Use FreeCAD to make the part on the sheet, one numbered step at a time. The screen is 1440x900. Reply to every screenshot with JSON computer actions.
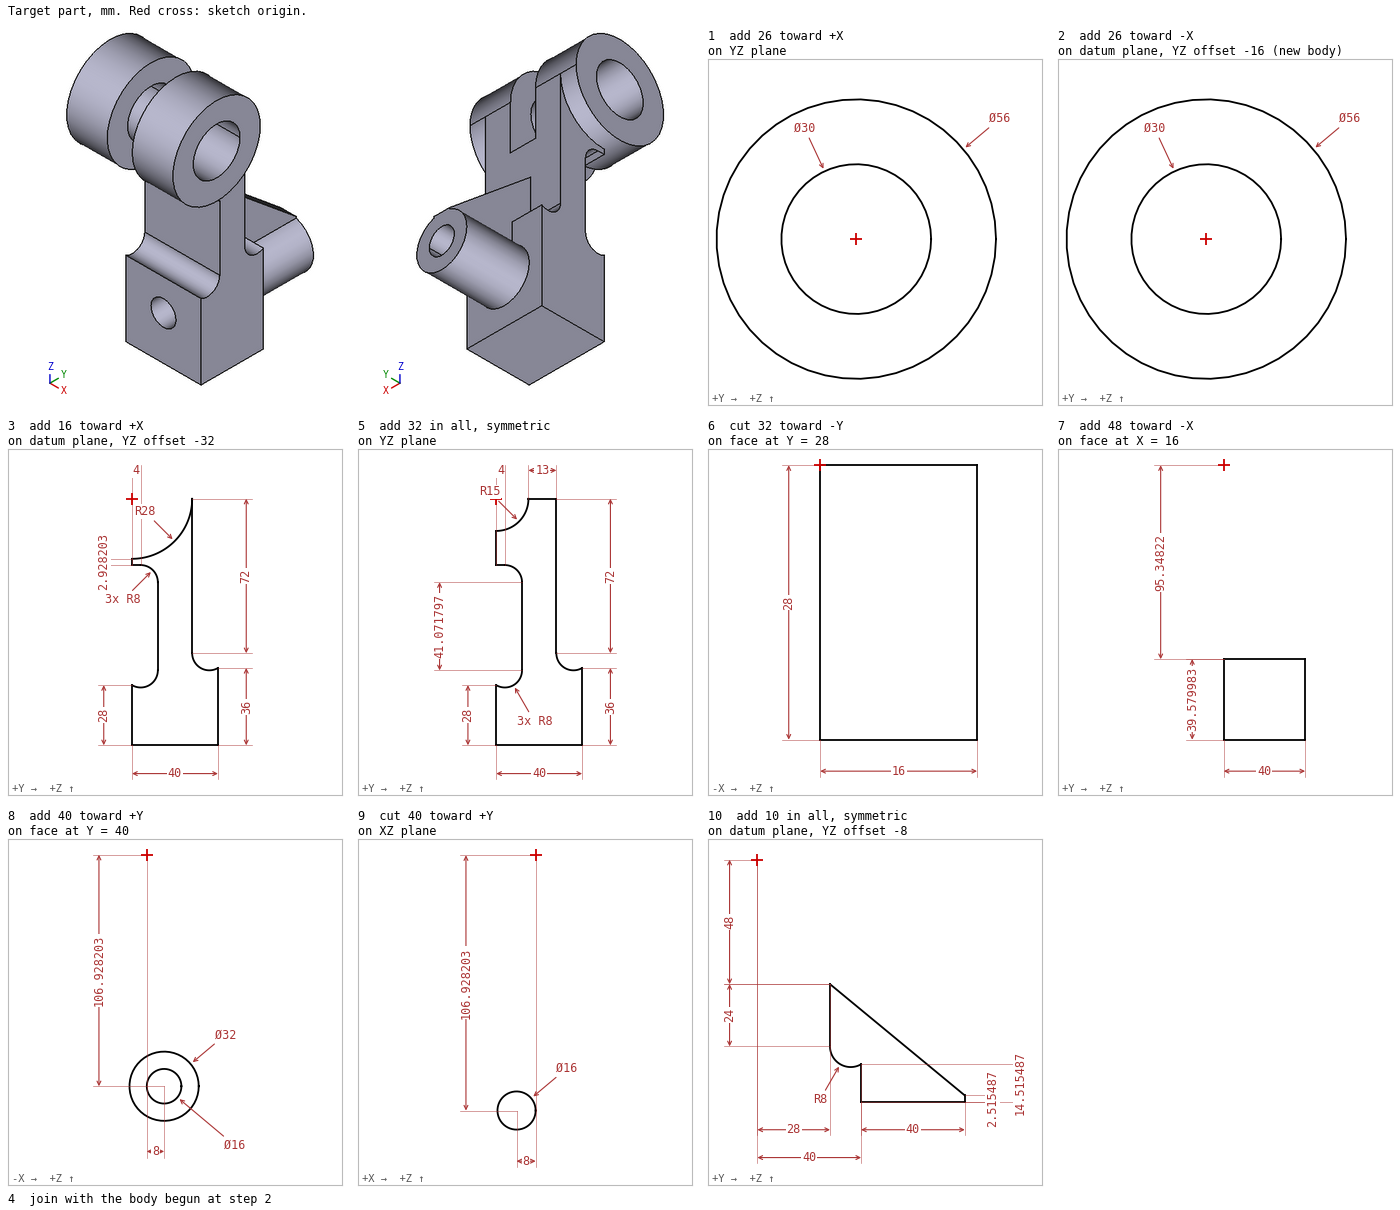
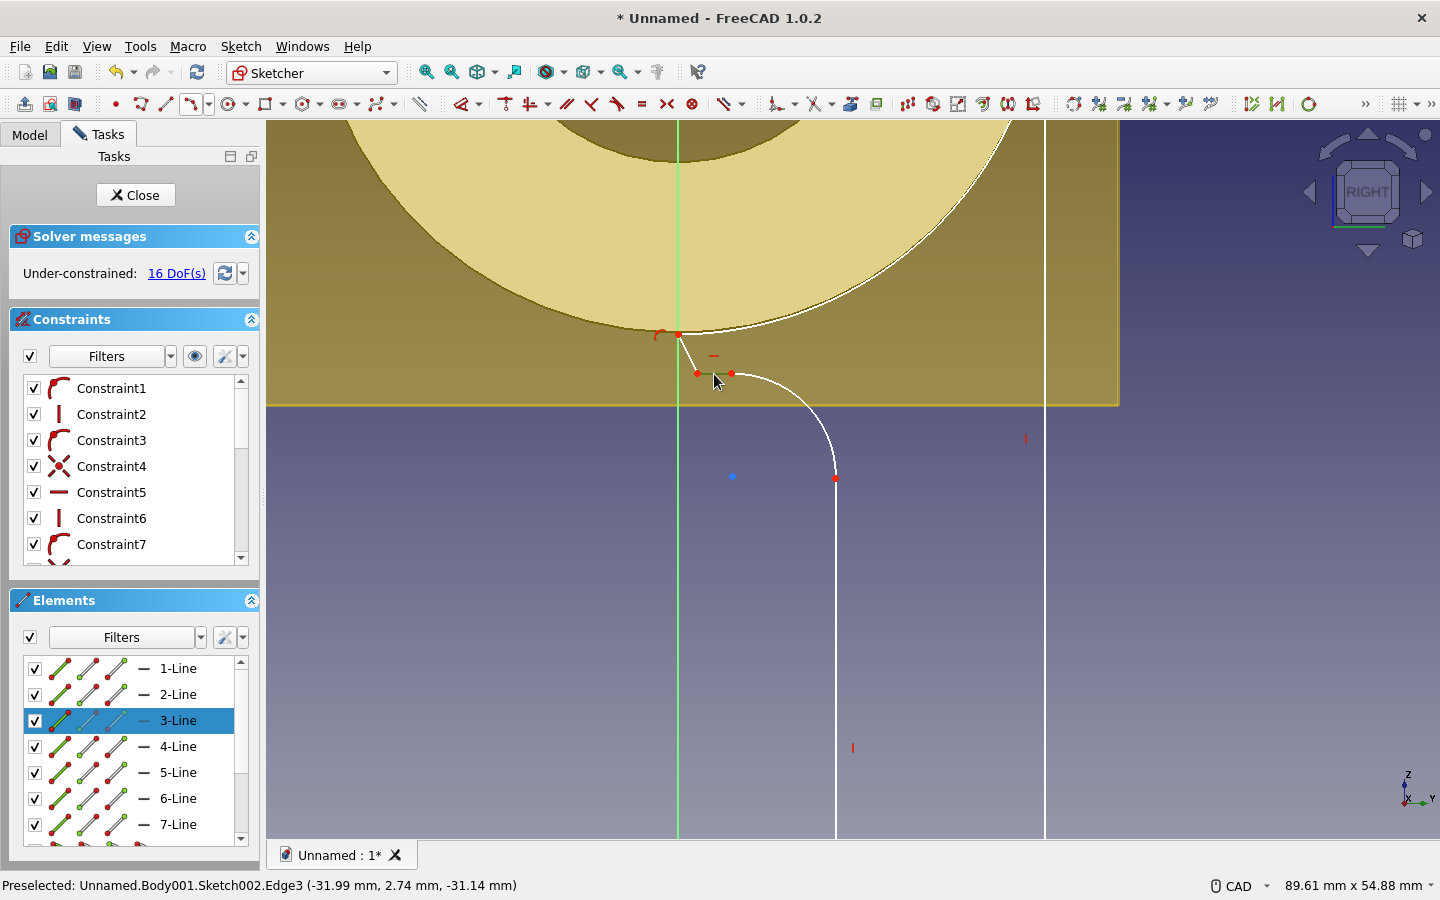
{"action": "left_click", "coordinate": [825, 431]}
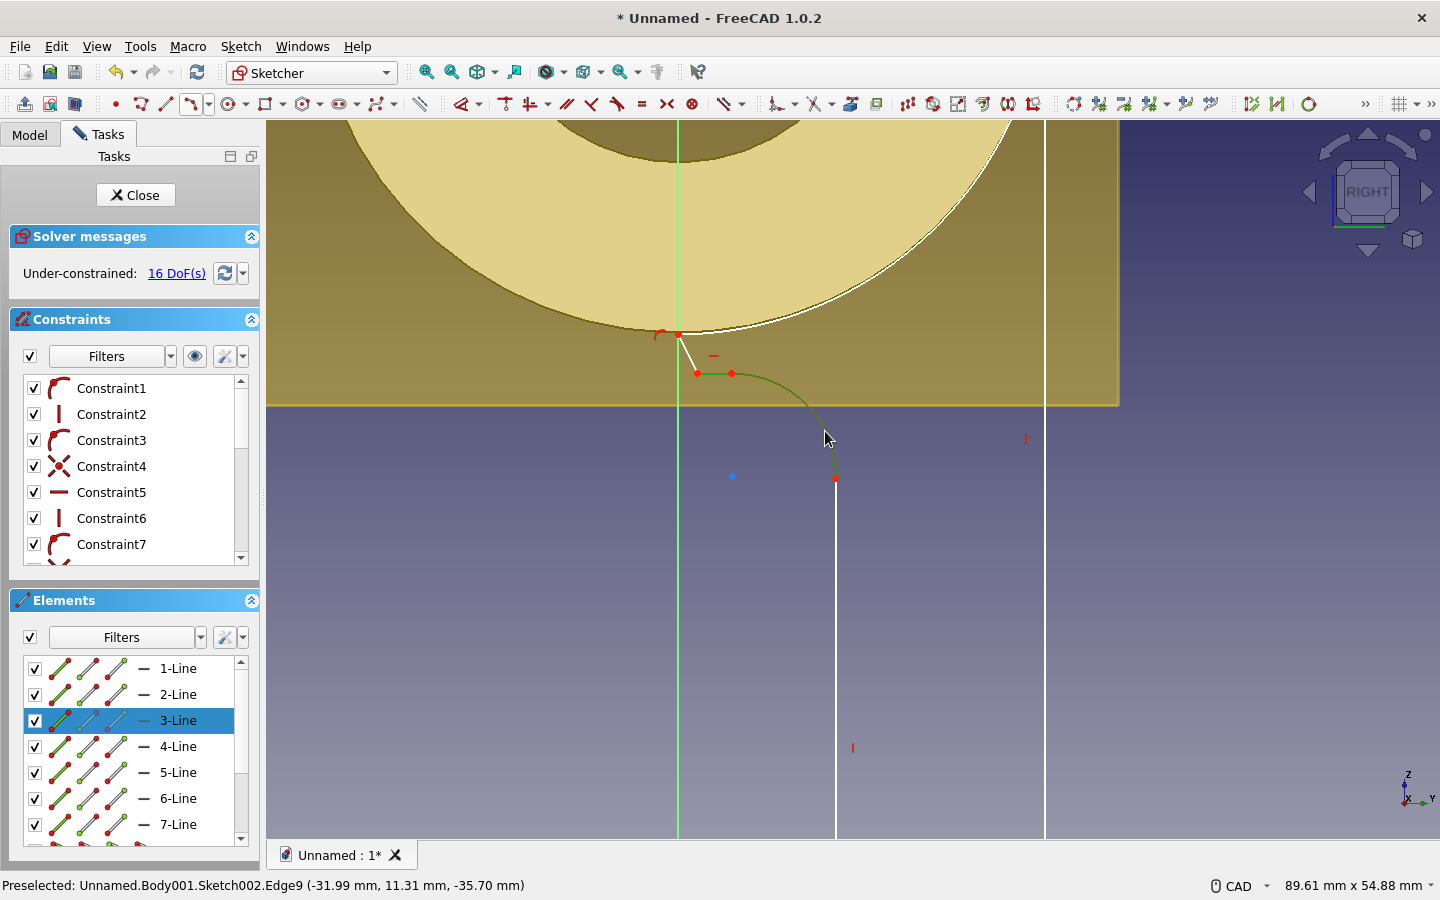
{"action": "left_click", "coordinate": [617, 104]}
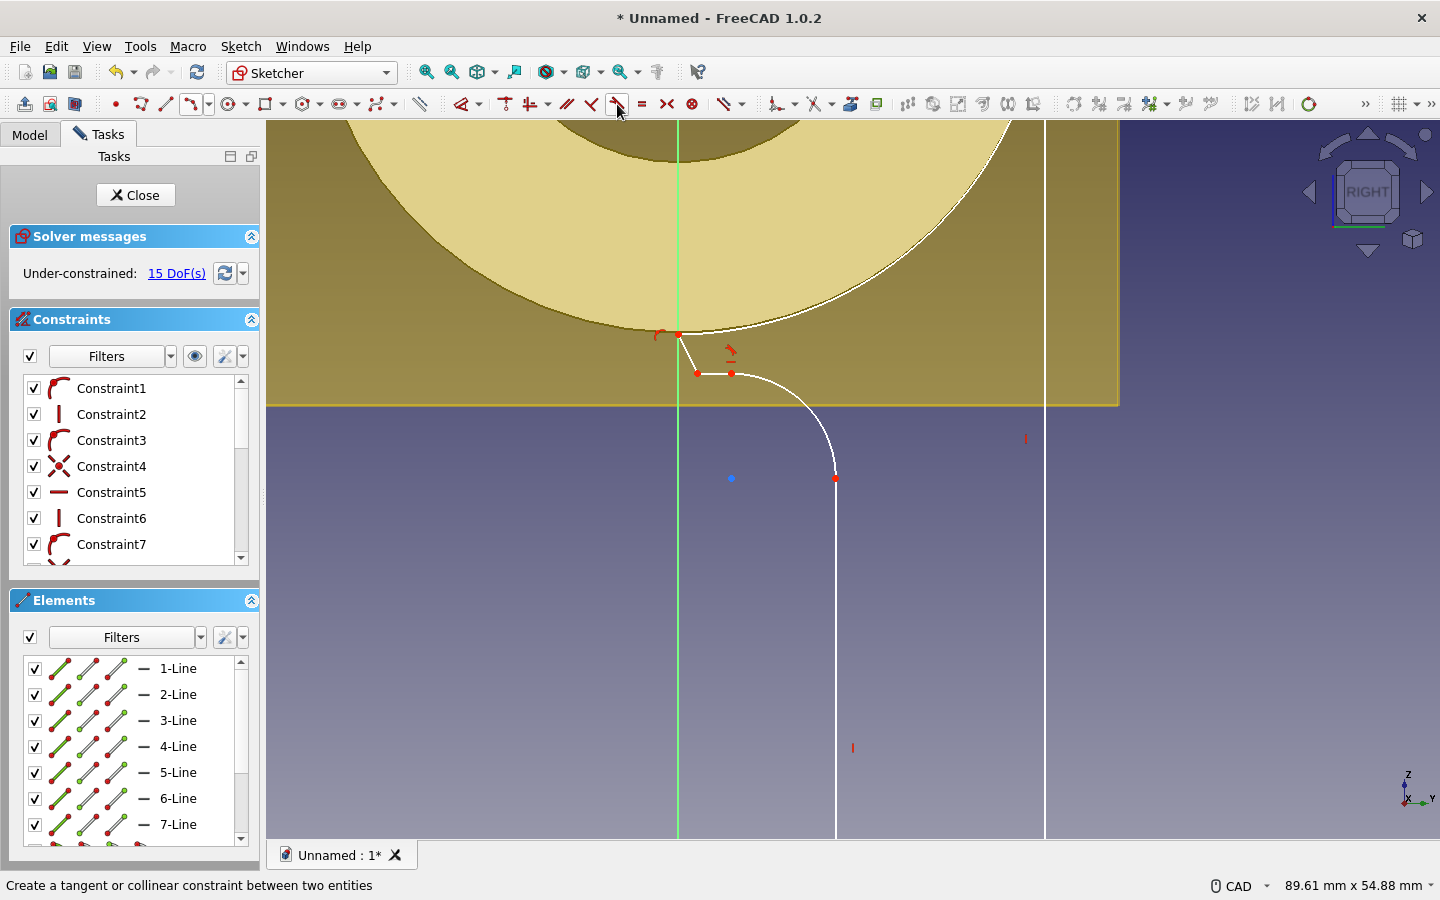
{"action": "left_click", "coordinate": [836, 640]}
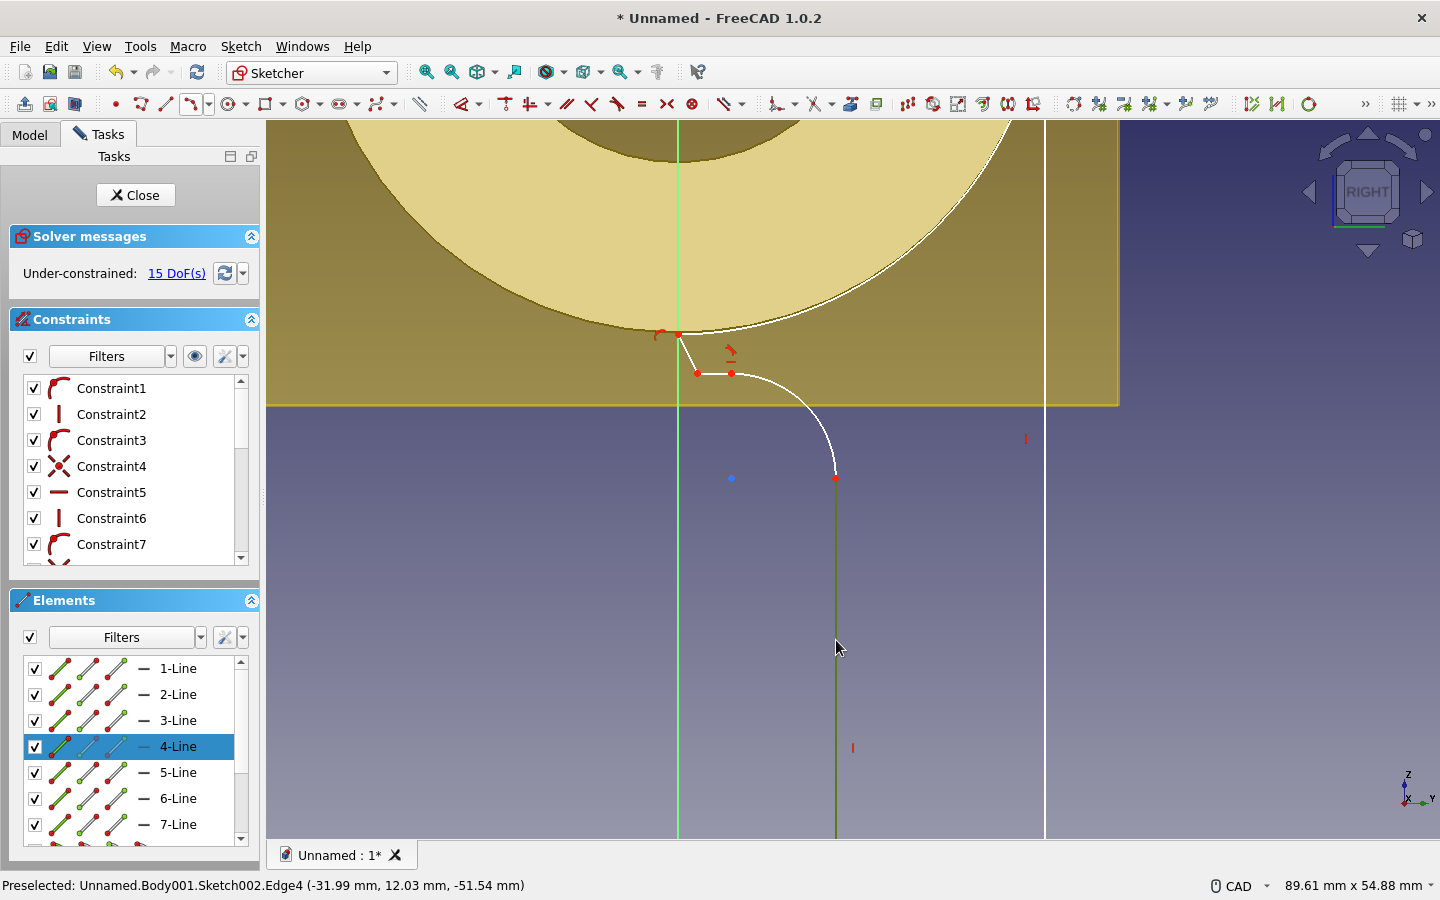
{"action": "left_click", "coordinate": [824, 431]}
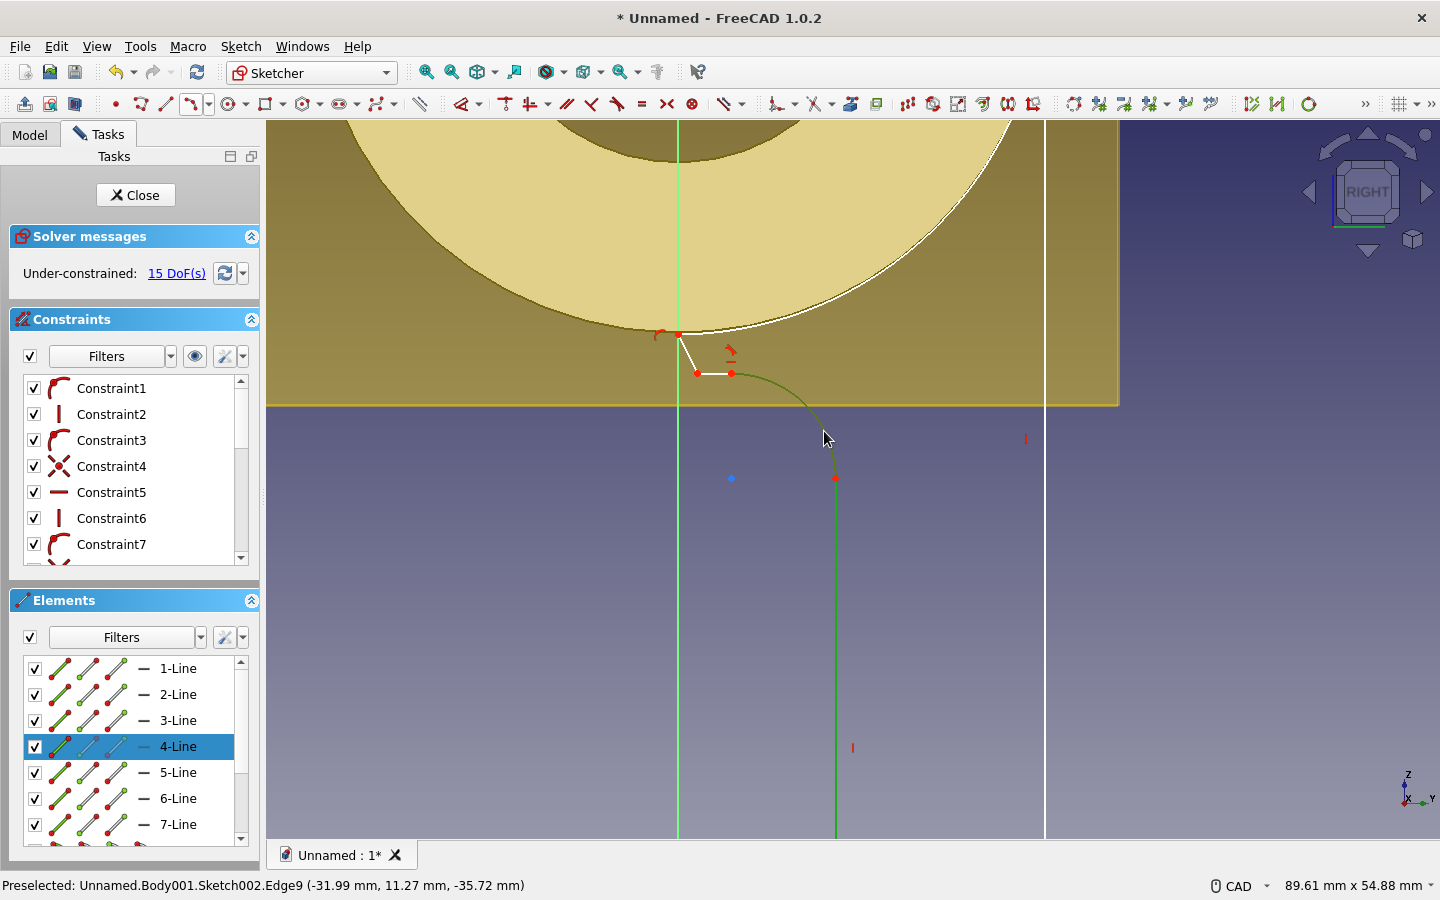
{"action": "key", "text": "t"}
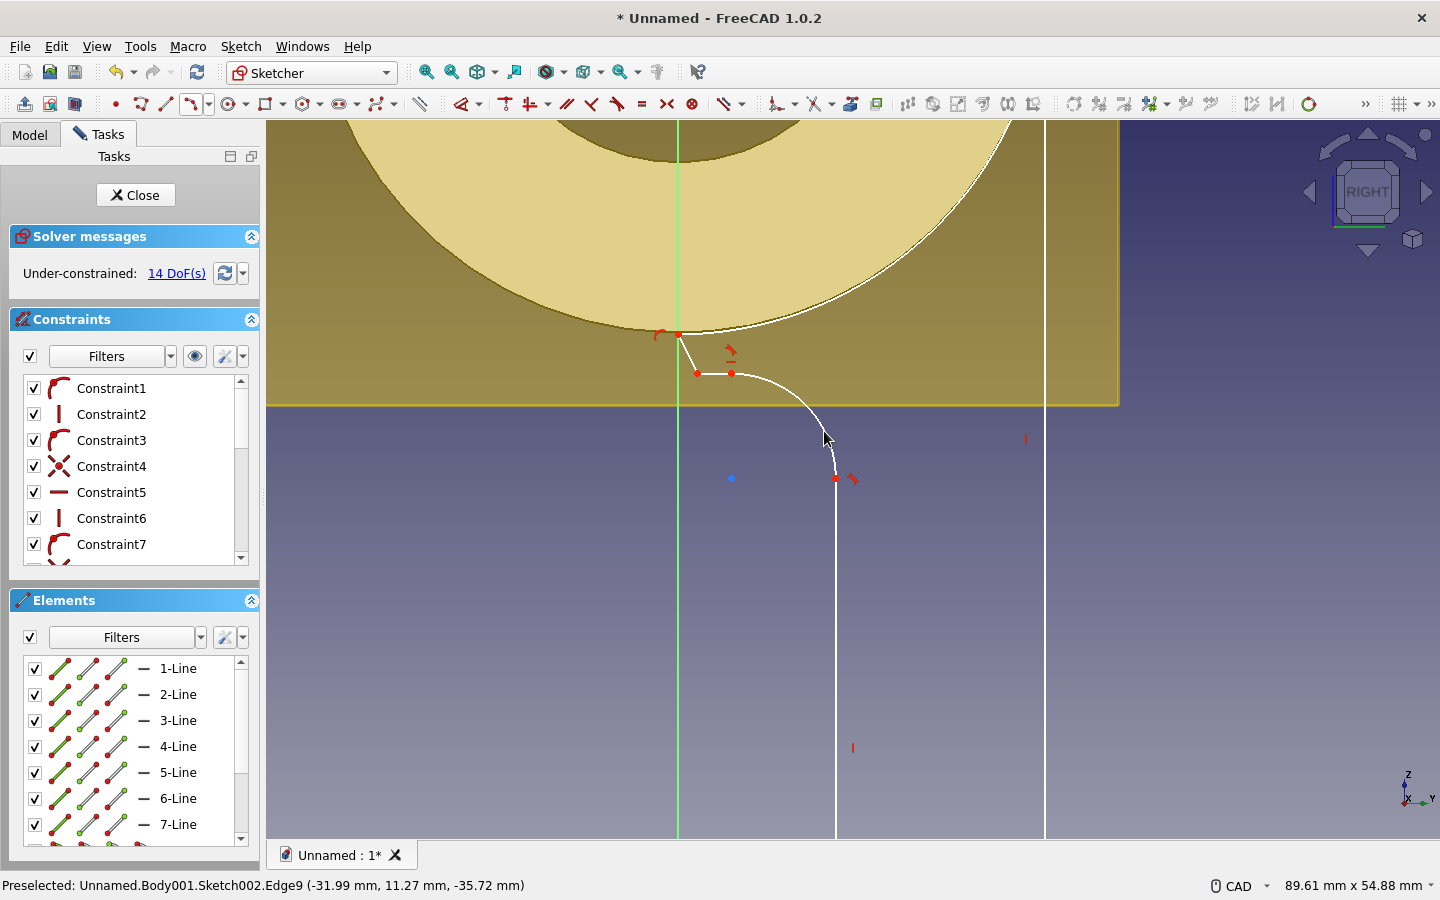
{"action": "left_click", "coordinate": [836, 640]}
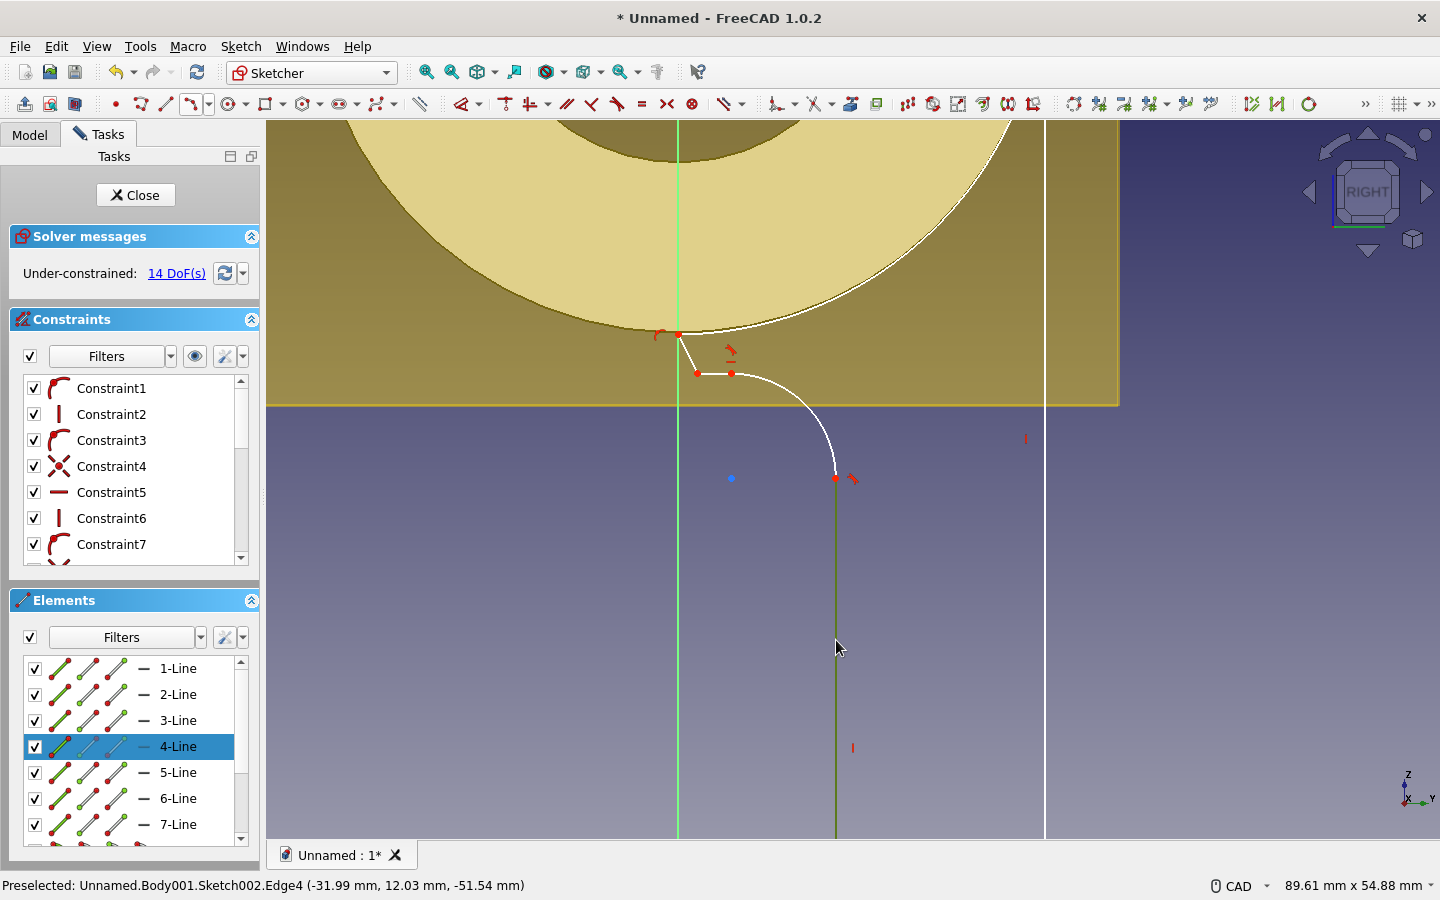
{"action": "scroll", "coordinate": [717, 376], "scroll_direction": "down", "scroll_amount": 6}